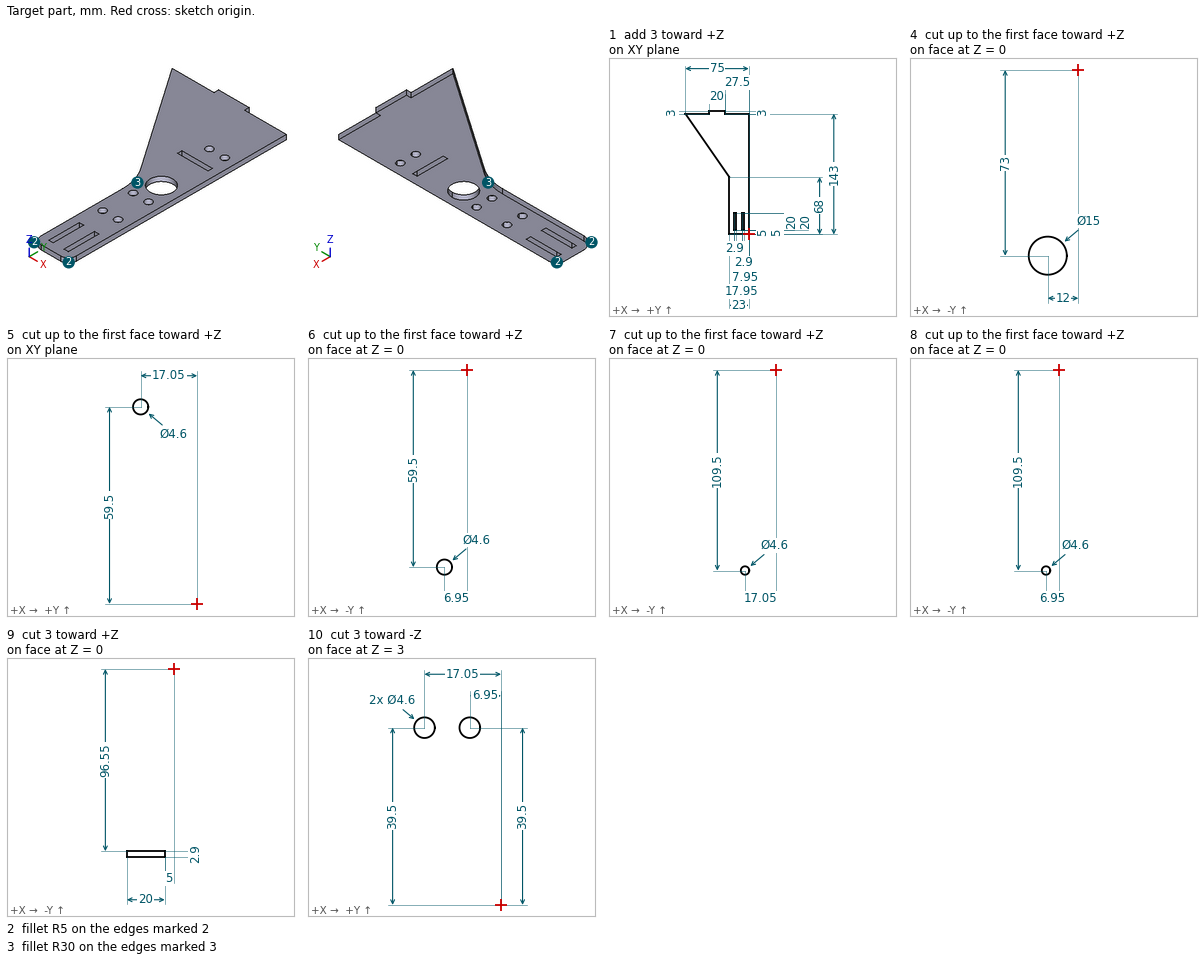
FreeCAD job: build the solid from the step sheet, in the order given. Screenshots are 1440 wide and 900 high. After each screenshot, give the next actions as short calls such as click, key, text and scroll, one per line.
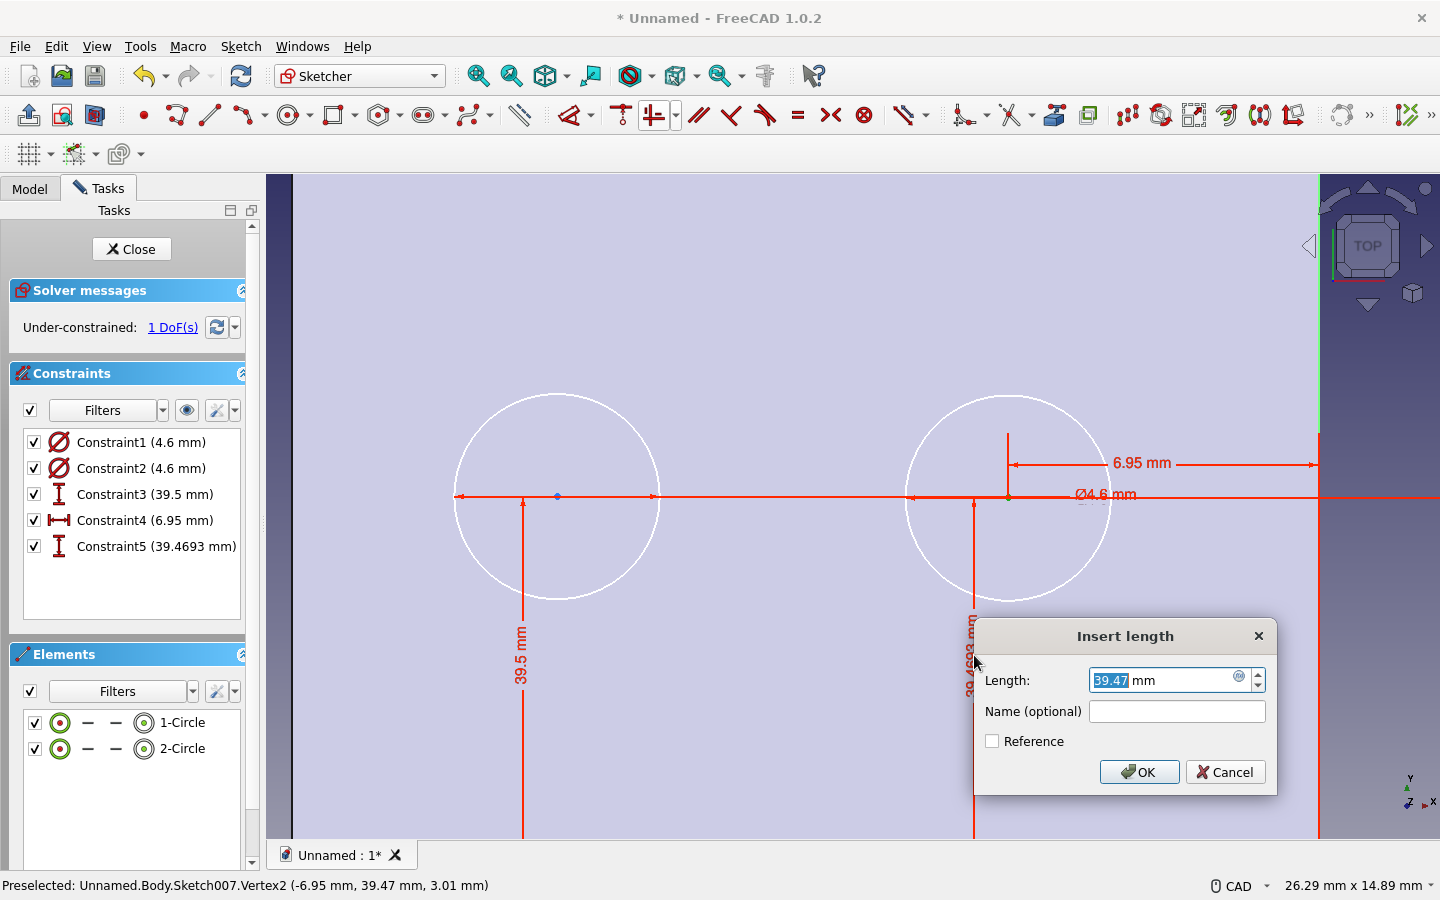
text(39.5)
key(Return)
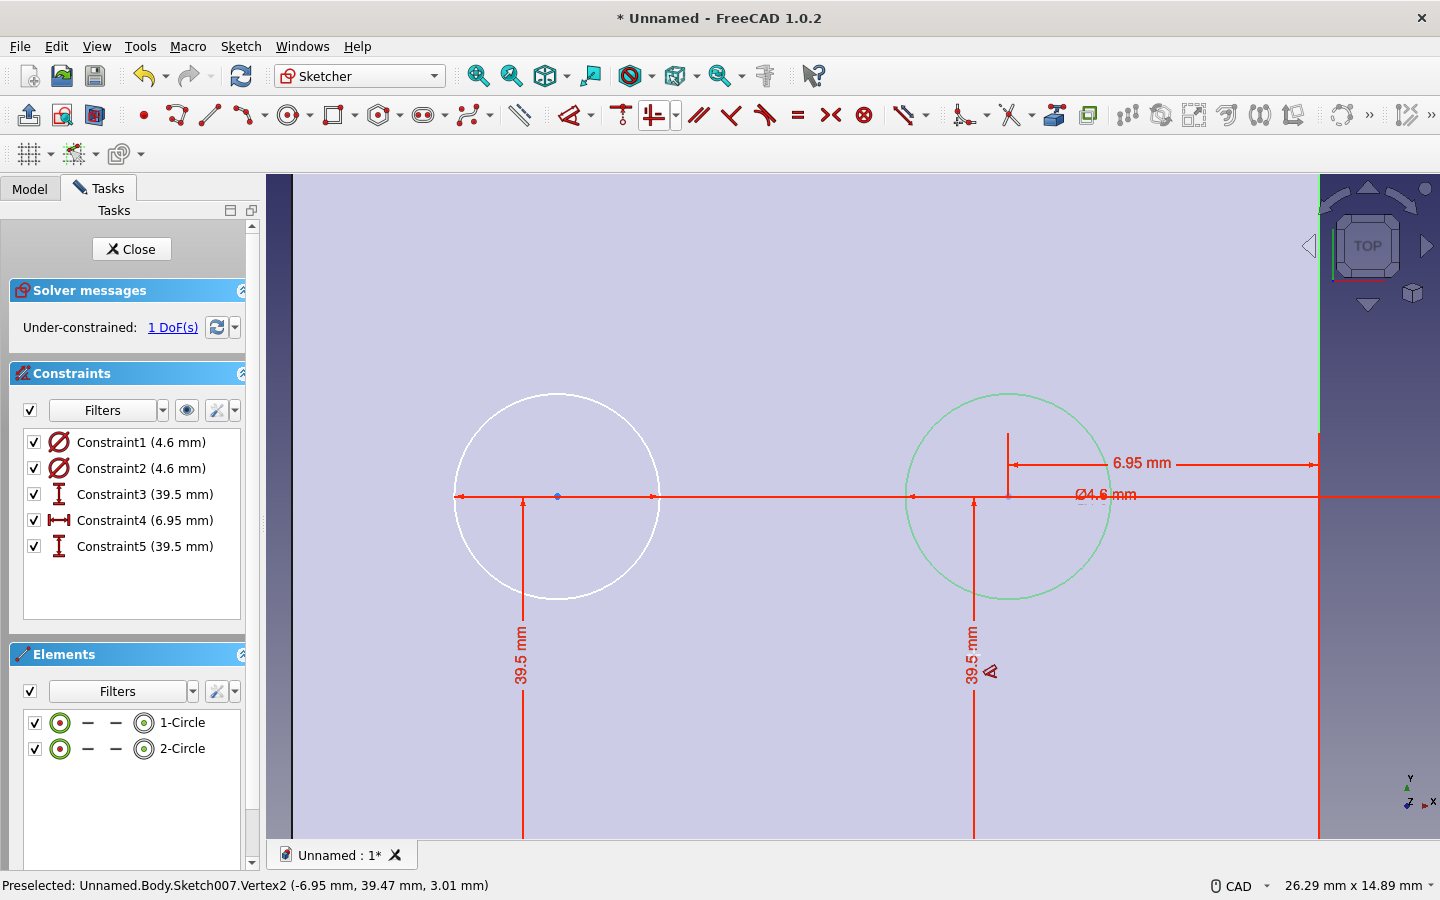
click(557, 497)
click(751, 463)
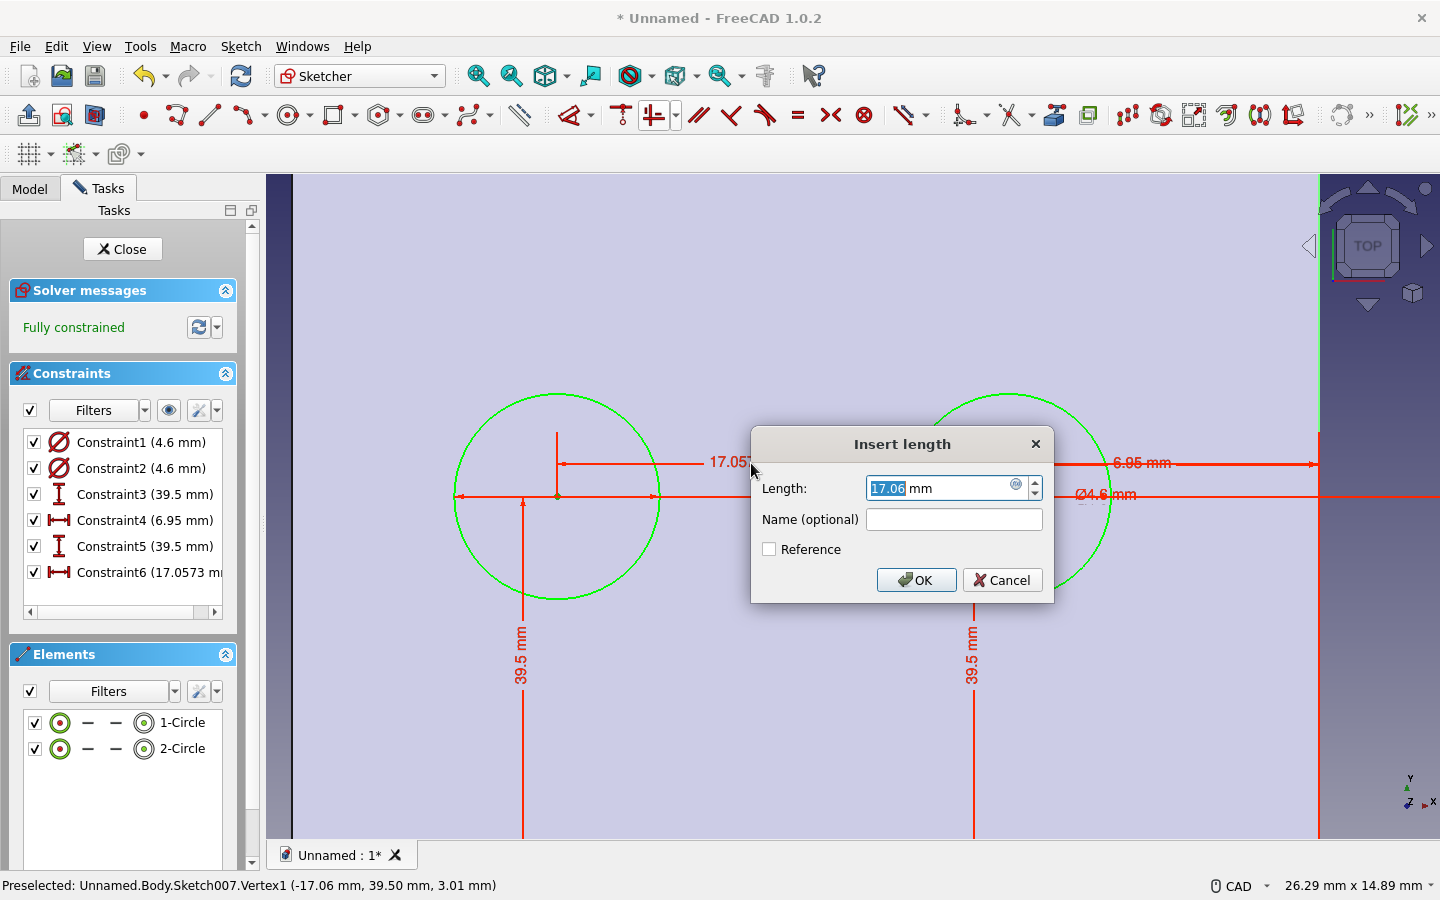
text(17.05)
key(Return)
key(Escape)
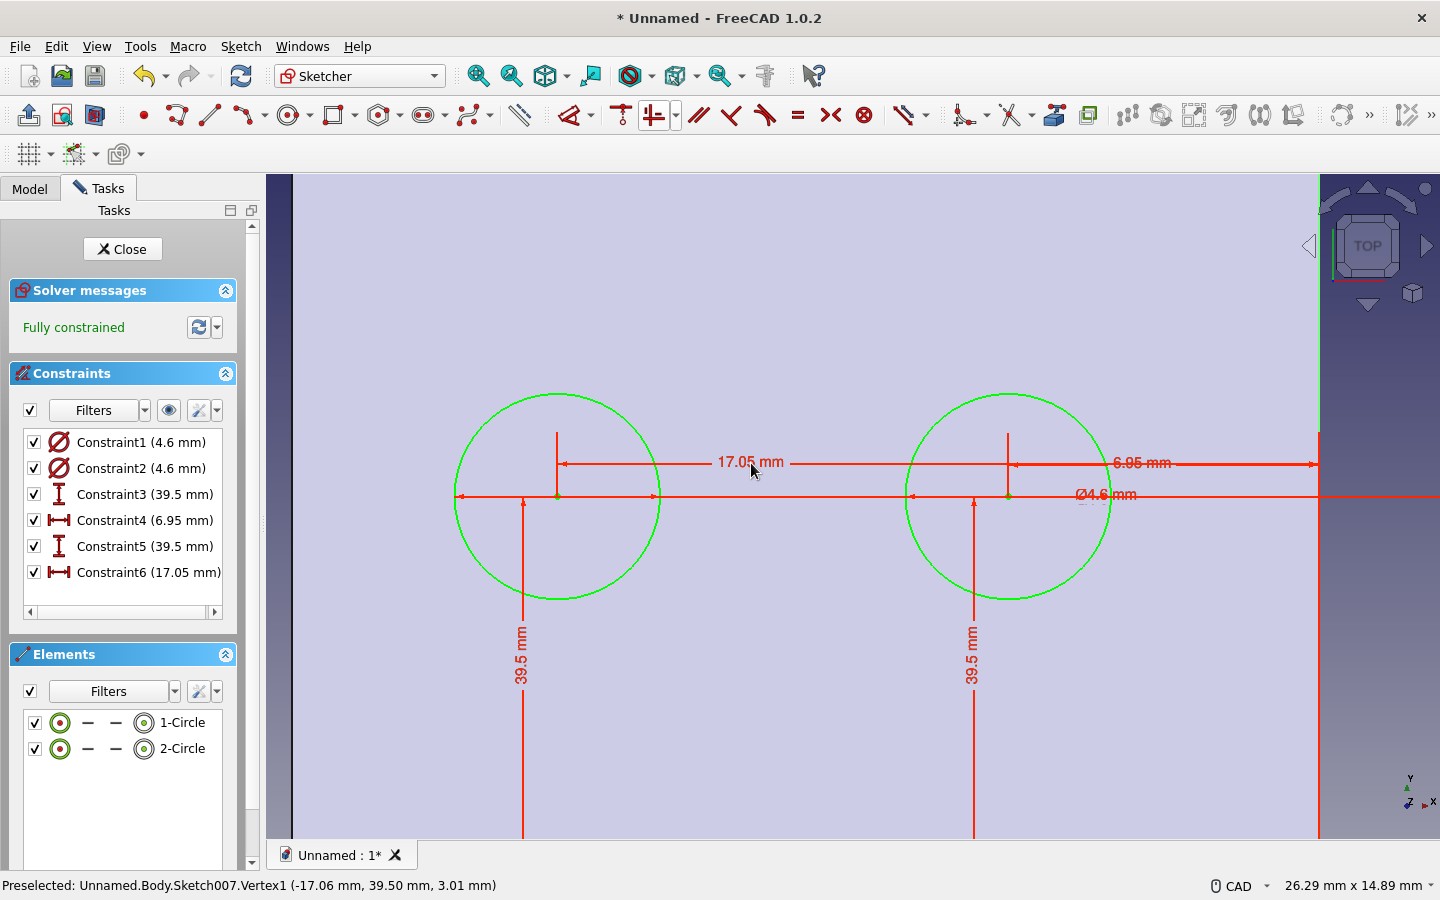
click(123, 249)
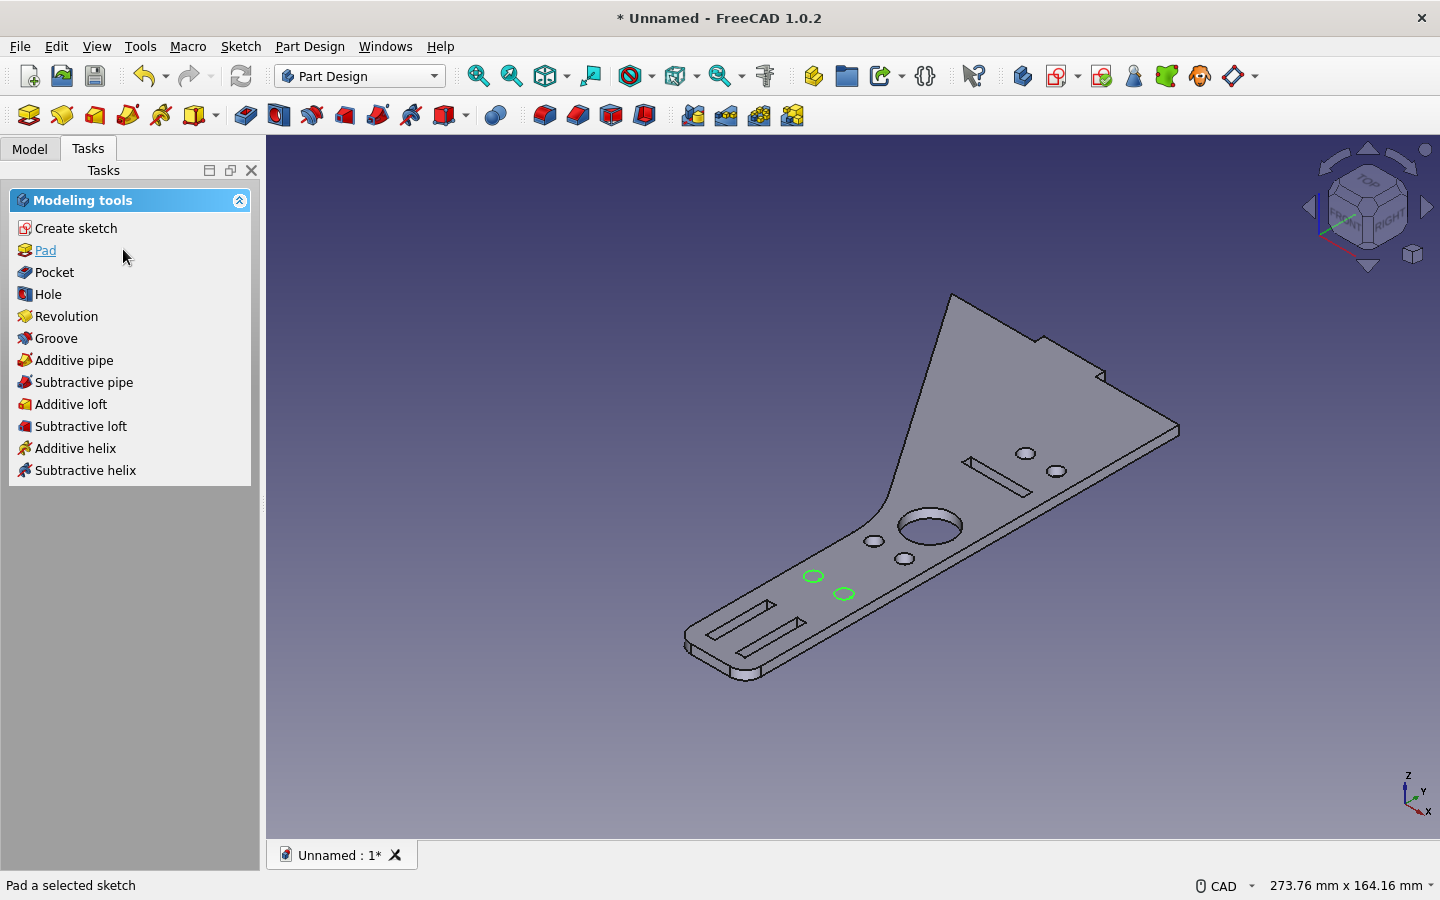
click(246, 116)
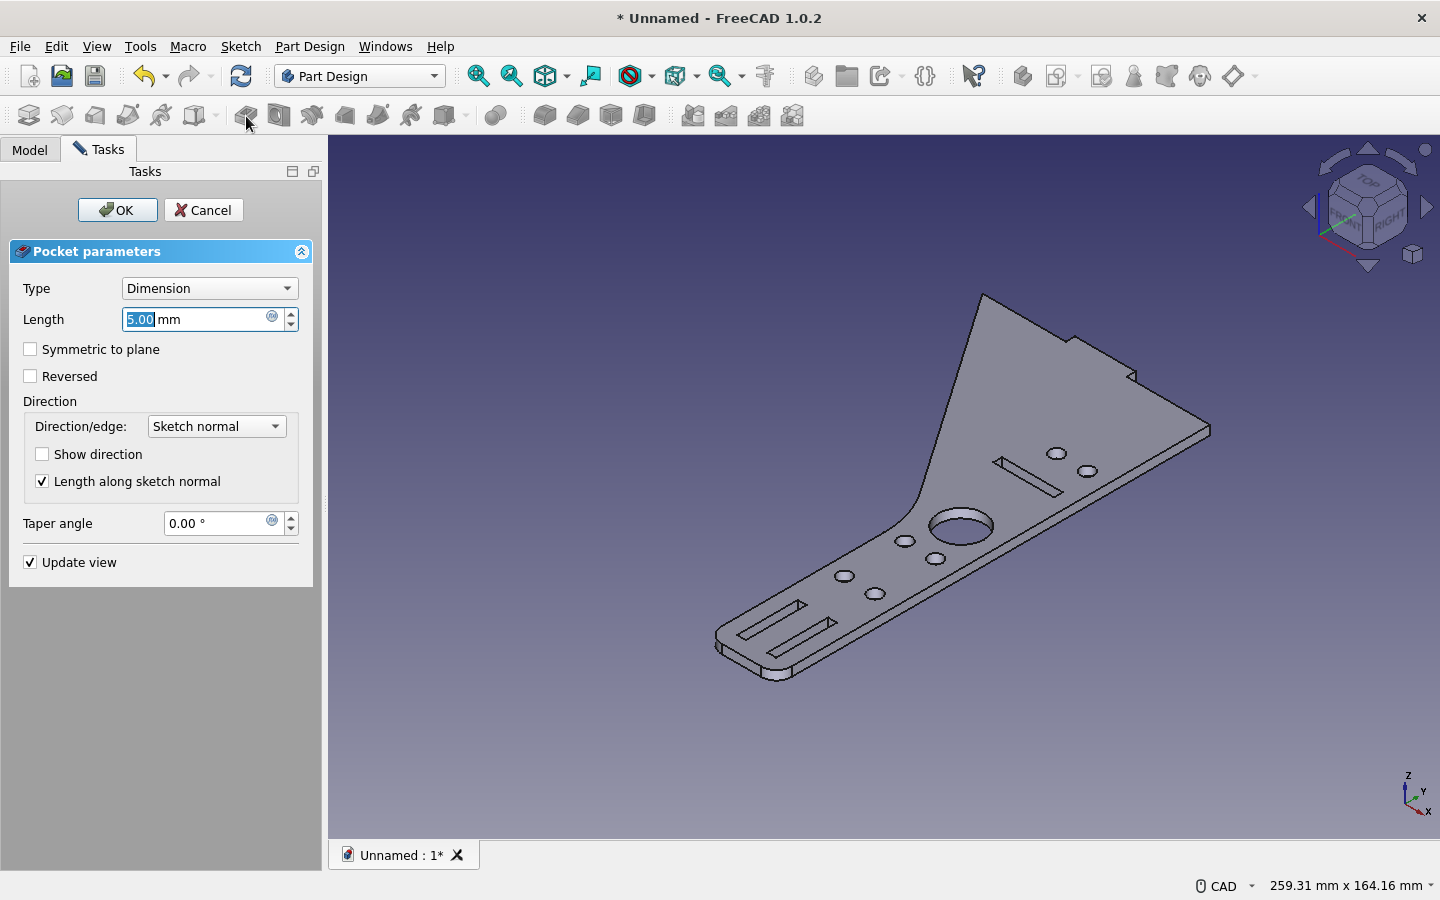
text(3)
key(Tab)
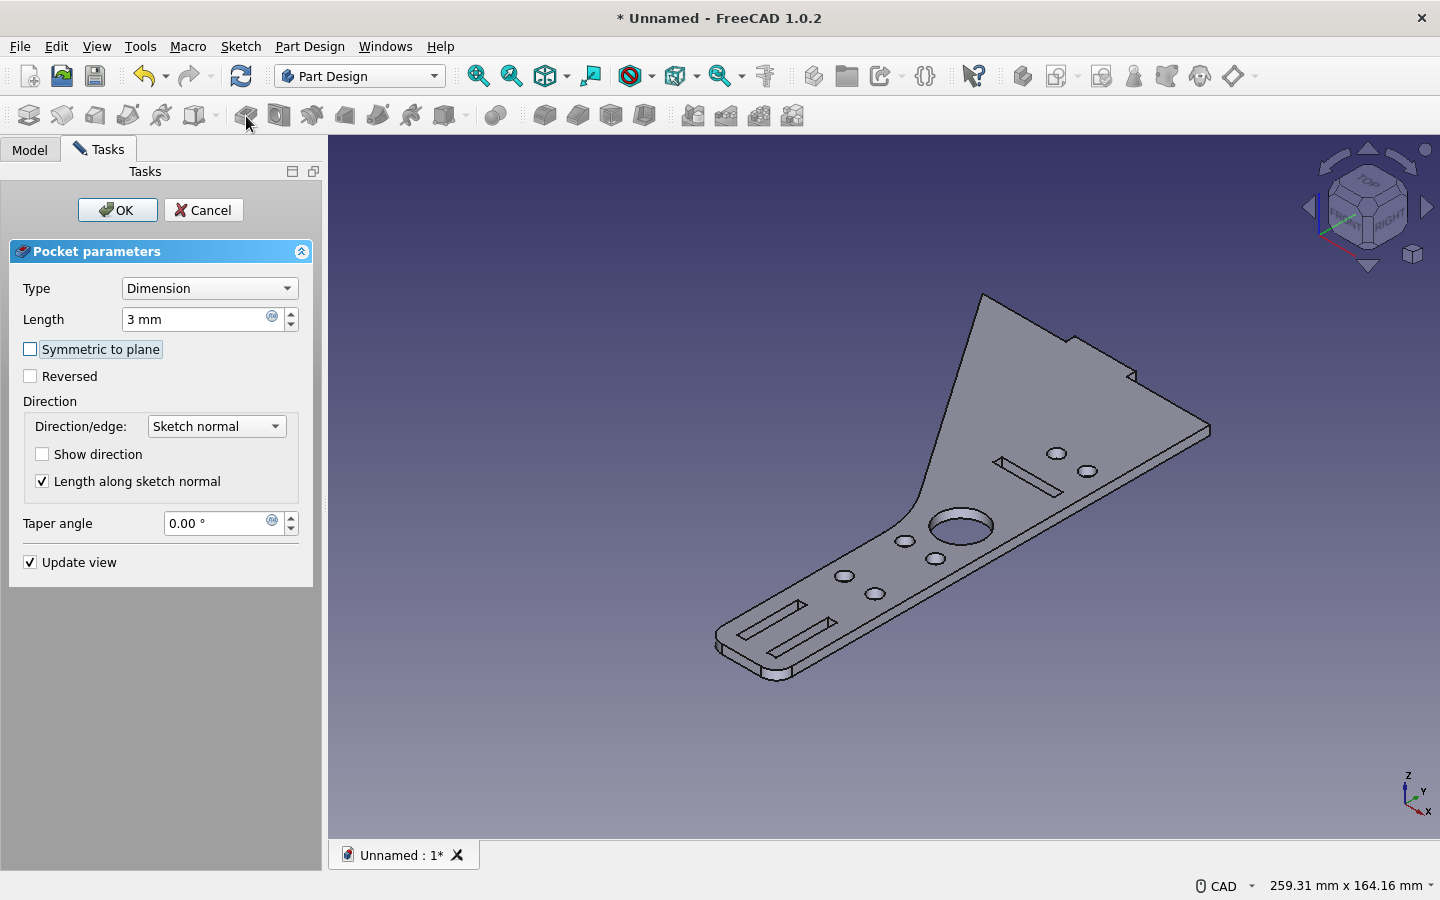
click(118, 210)